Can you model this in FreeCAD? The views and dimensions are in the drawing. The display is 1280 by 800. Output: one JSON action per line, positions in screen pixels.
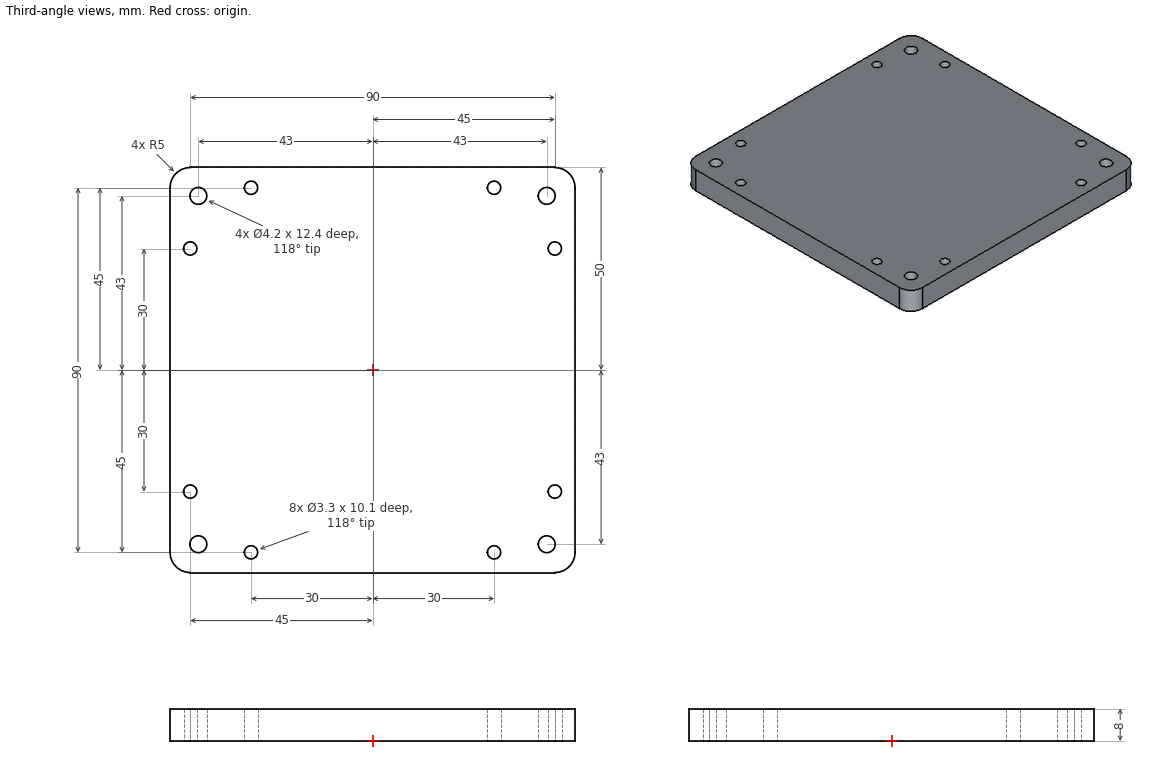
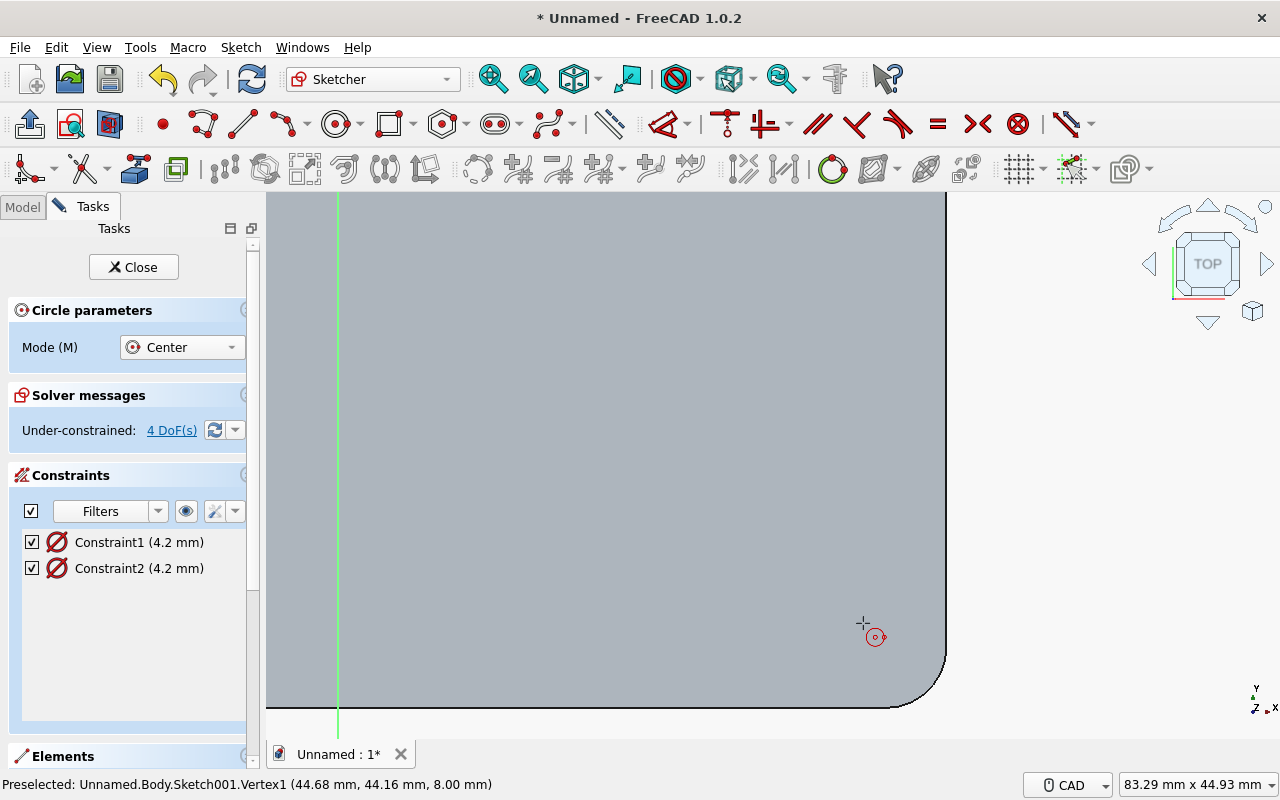
{"action": "left_click", "coordinate": [861, 623]}
{"action": "mouse_move", "coordinate": [879, 605]}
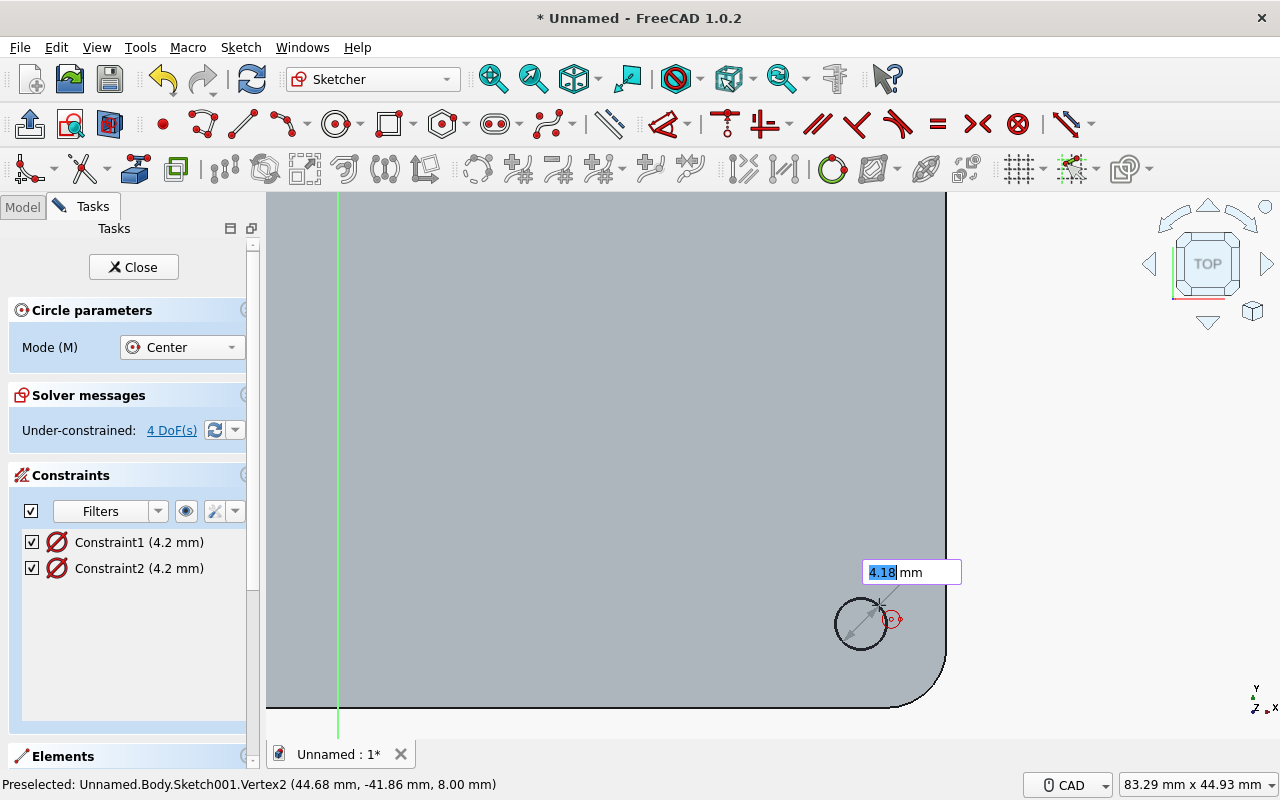
{"action": "type", "text": "4.2"}
{"action": "key", "text": "Return"}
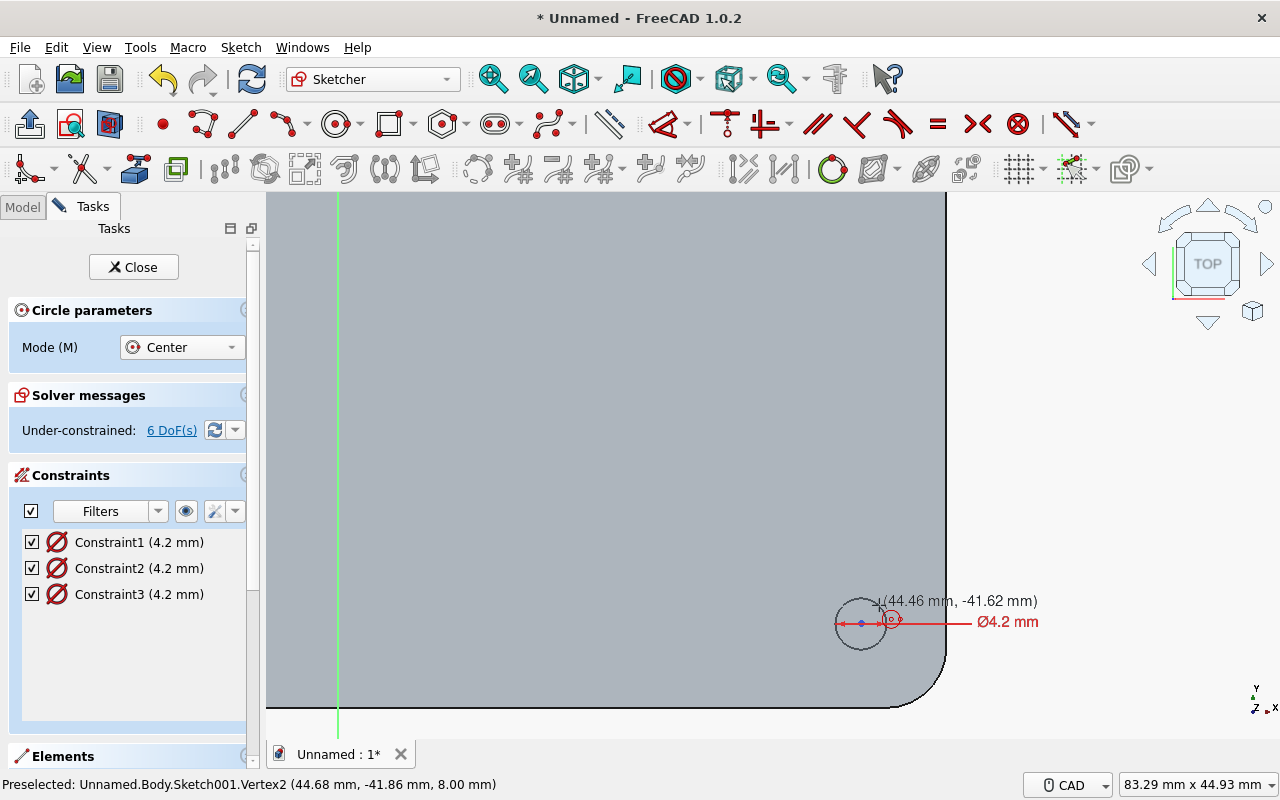
{"action": "scroll", "coordinate": [863, 623], "scroll_direction": "down", "scroll_amount": 6}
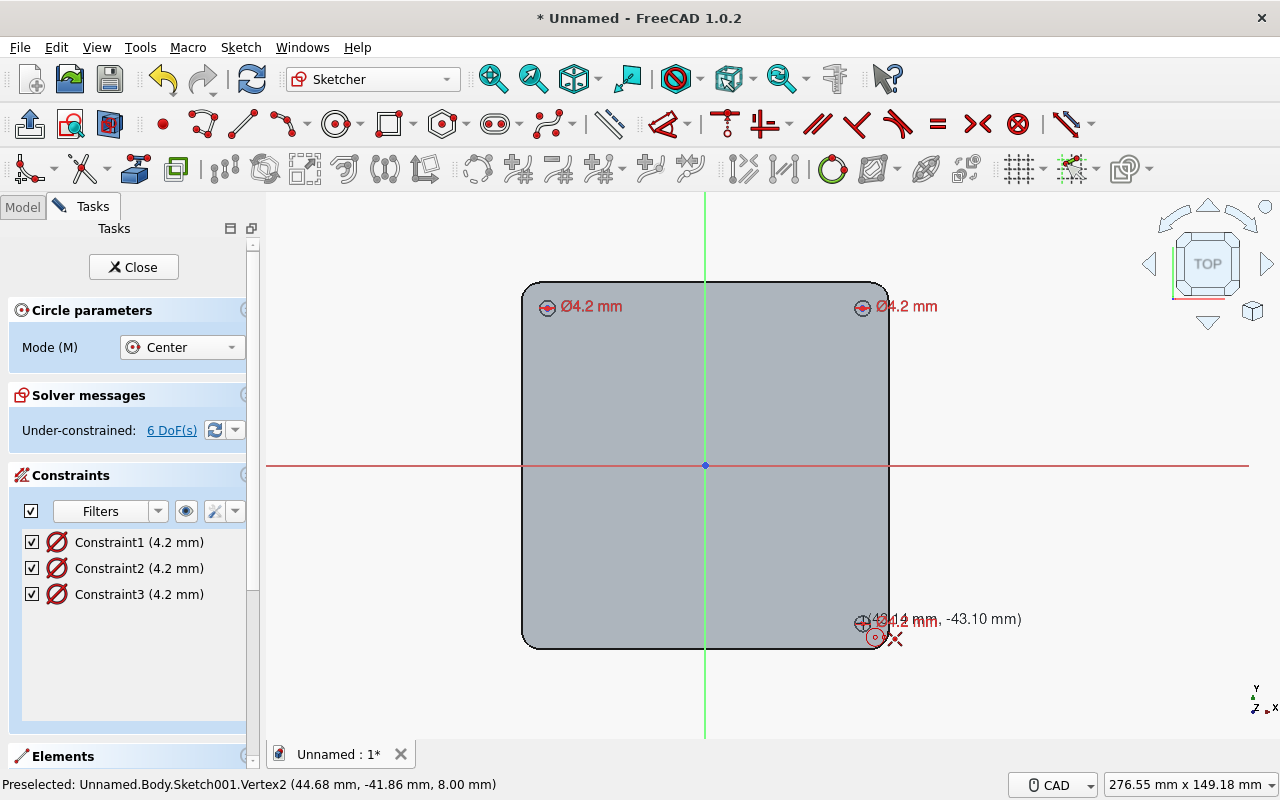
{"action": "scroll", "coordinate": [548, 623], "scroll_direction": "up", "scroll_amount": 6}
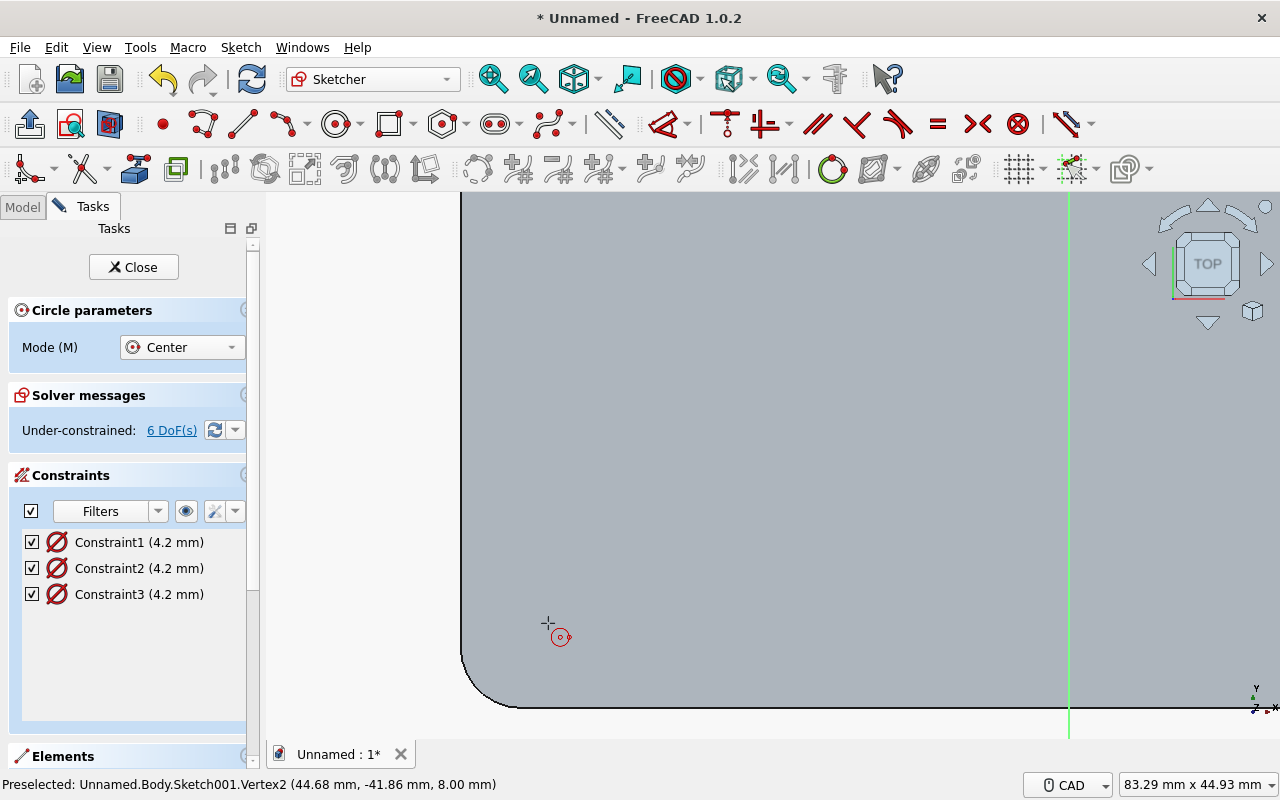
{"action": "left_click", "coordinate": [546, 623]}
{"action": "mouse_move", "coordinate": [564, 605]}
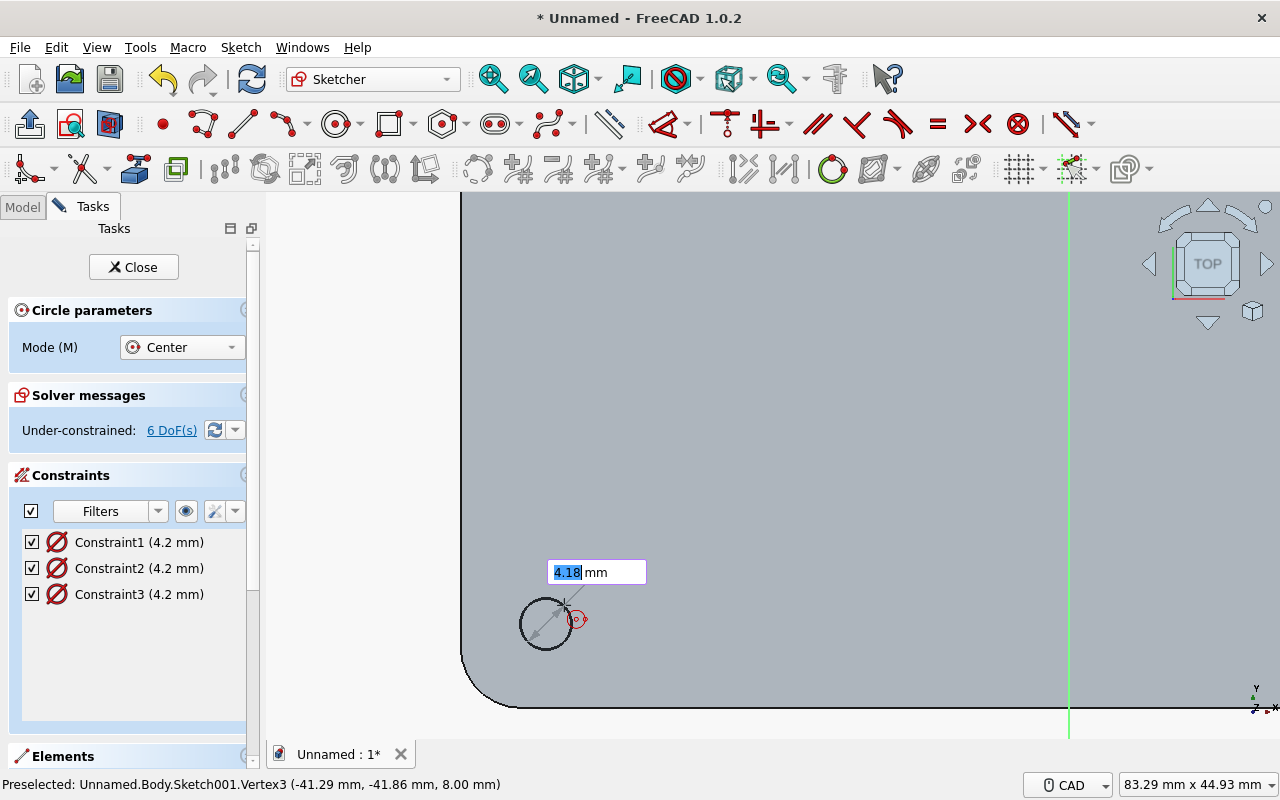
{"action": "type", "text": "4.2"}
{"action": "key", "text": "Return"}
{"action": "key", "text": "Escape"}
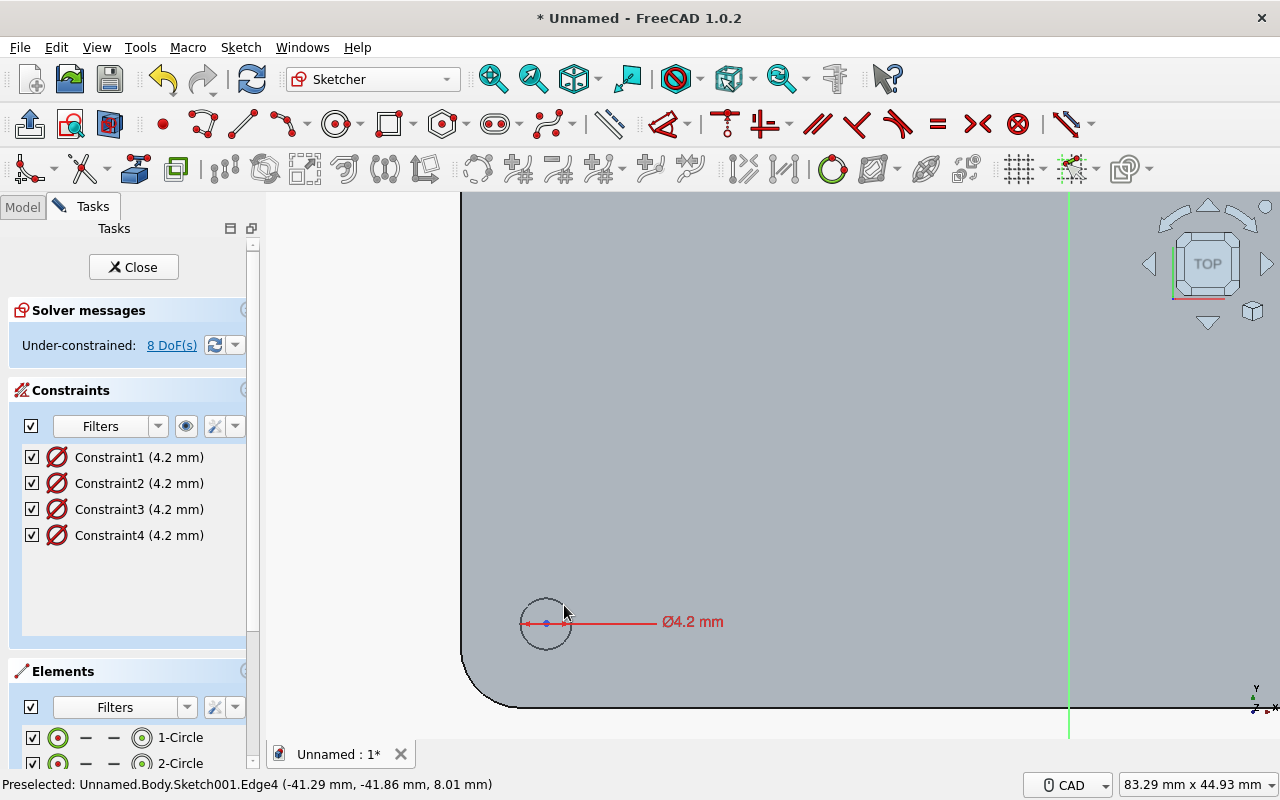
{"action": "scroll", "coordinate": [547, 623], "scroll_direction": "down", "scroll_amount": 6}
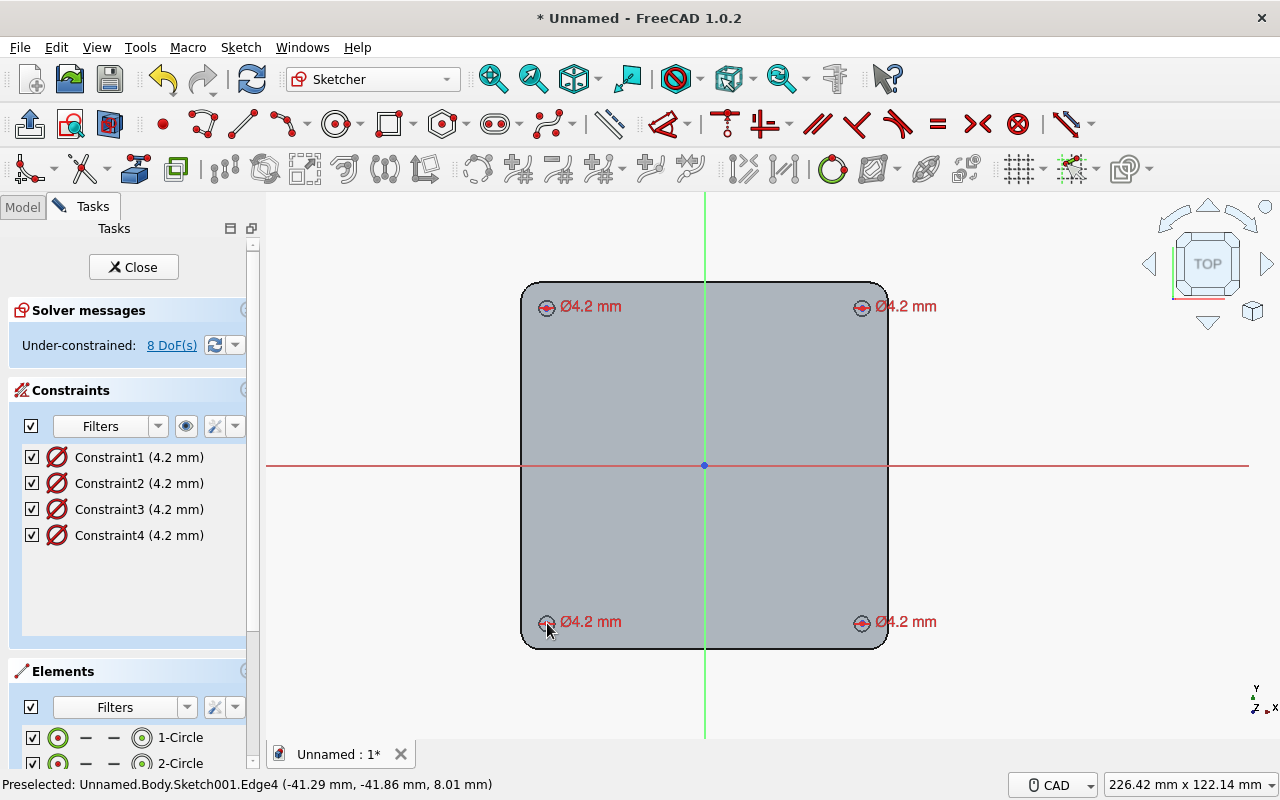
{"action": "left_click", "coordinate": [547, 308]}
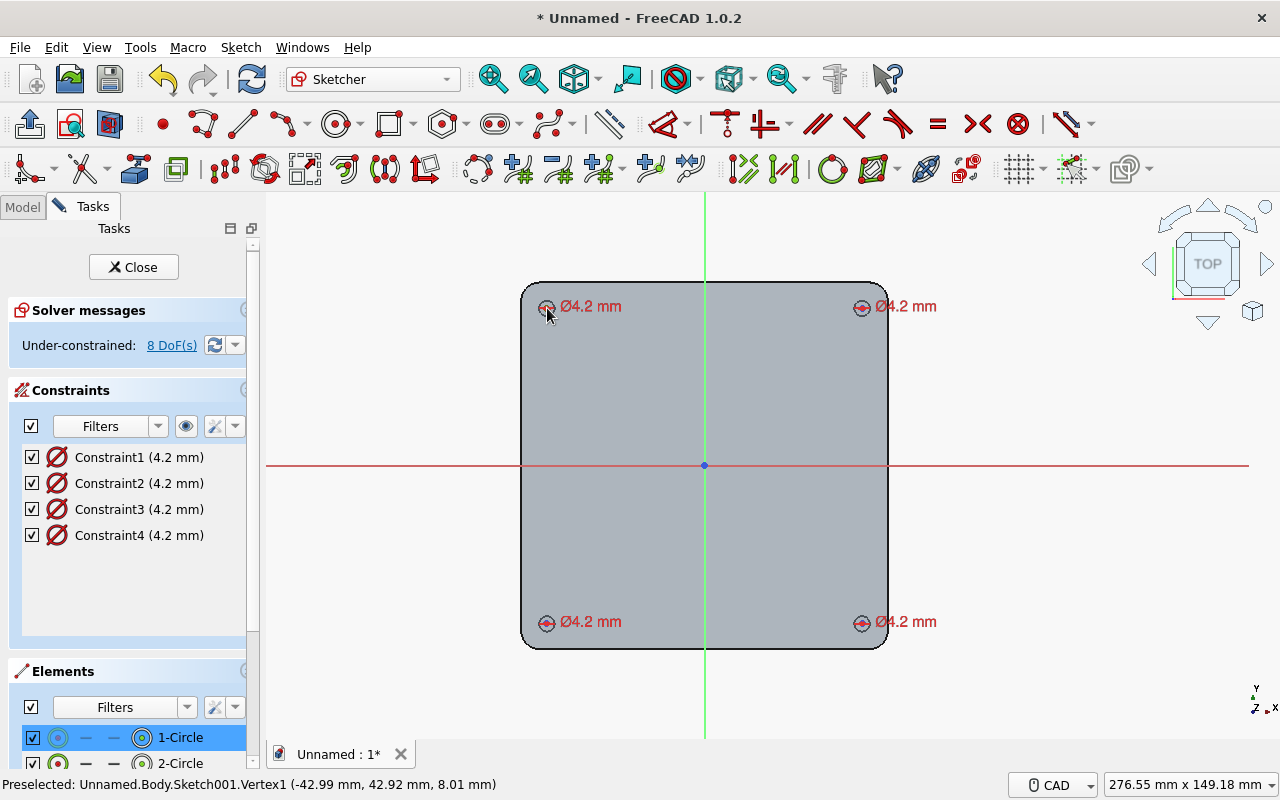
{"action": "left_click", "coordinate": [862, 308]}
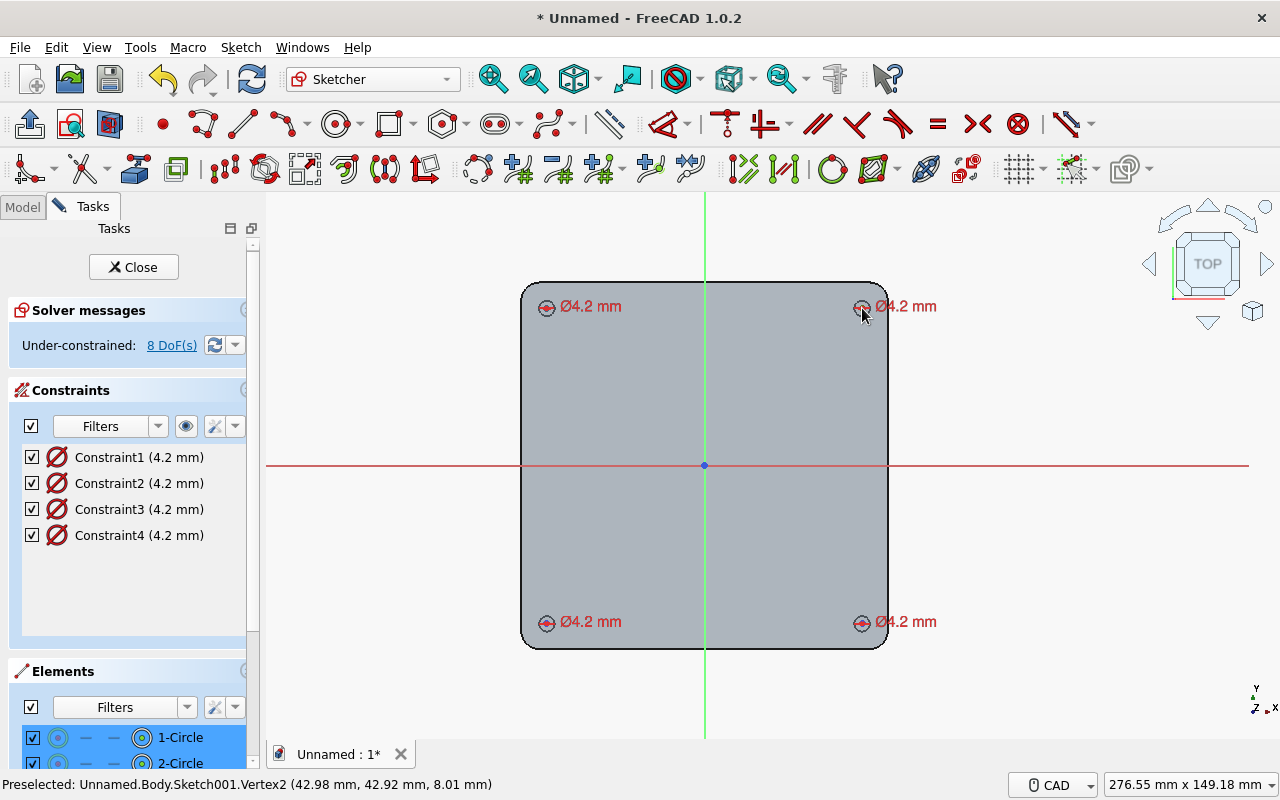
{"action": "key", "text": "h"}